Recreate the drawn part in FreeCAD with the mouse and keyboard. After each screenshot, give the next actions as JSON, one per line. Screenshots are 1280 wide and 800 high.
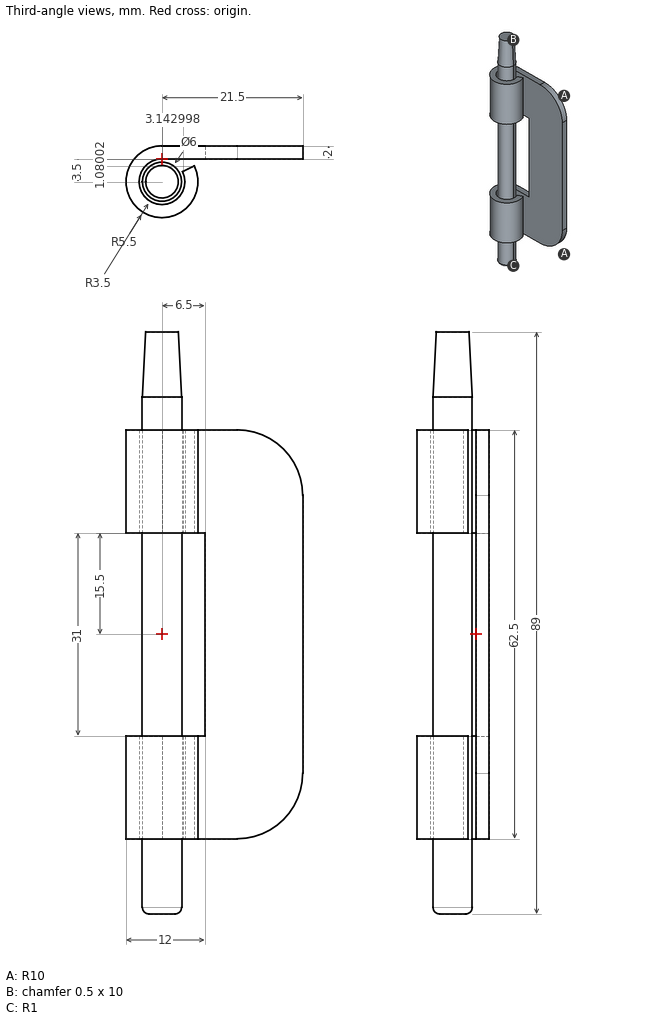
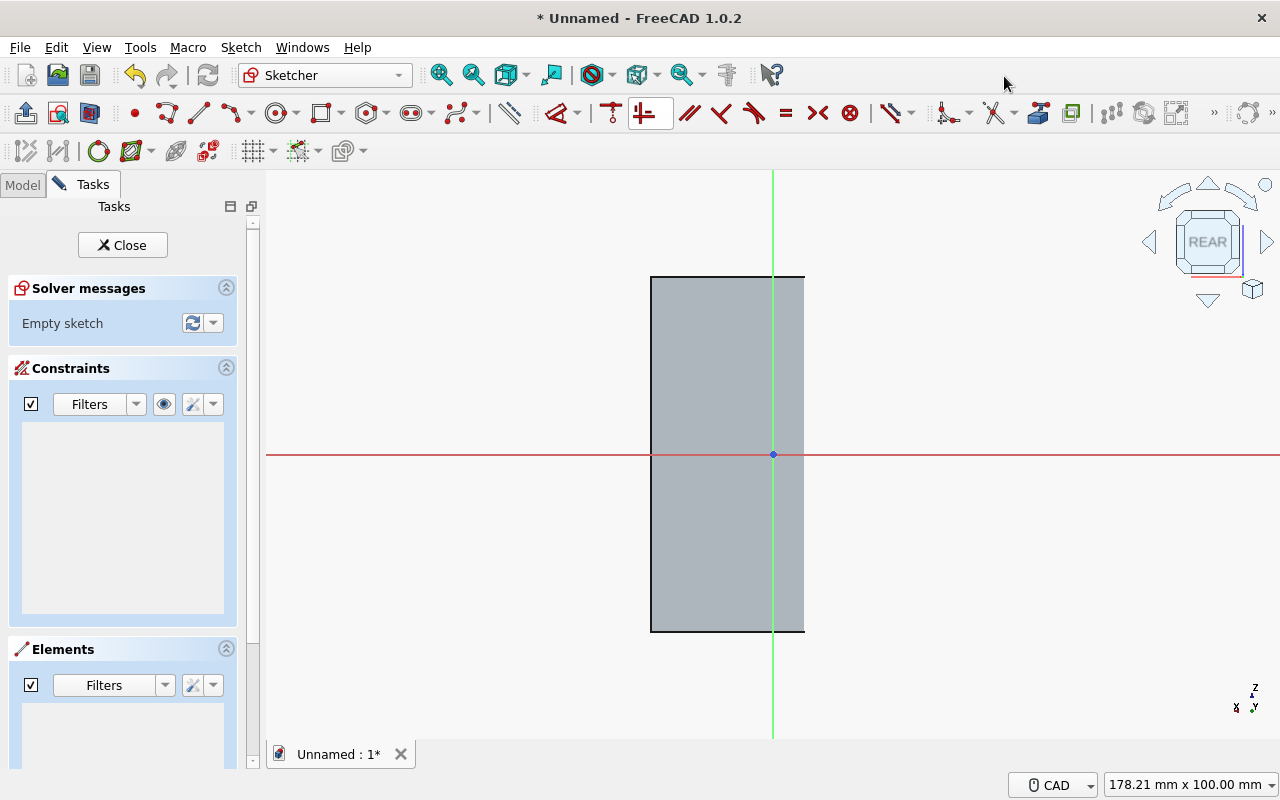
{"action": "scroll", "coordinate": [824, 454], "scroll_direction": "up", "scroll_amount": 4}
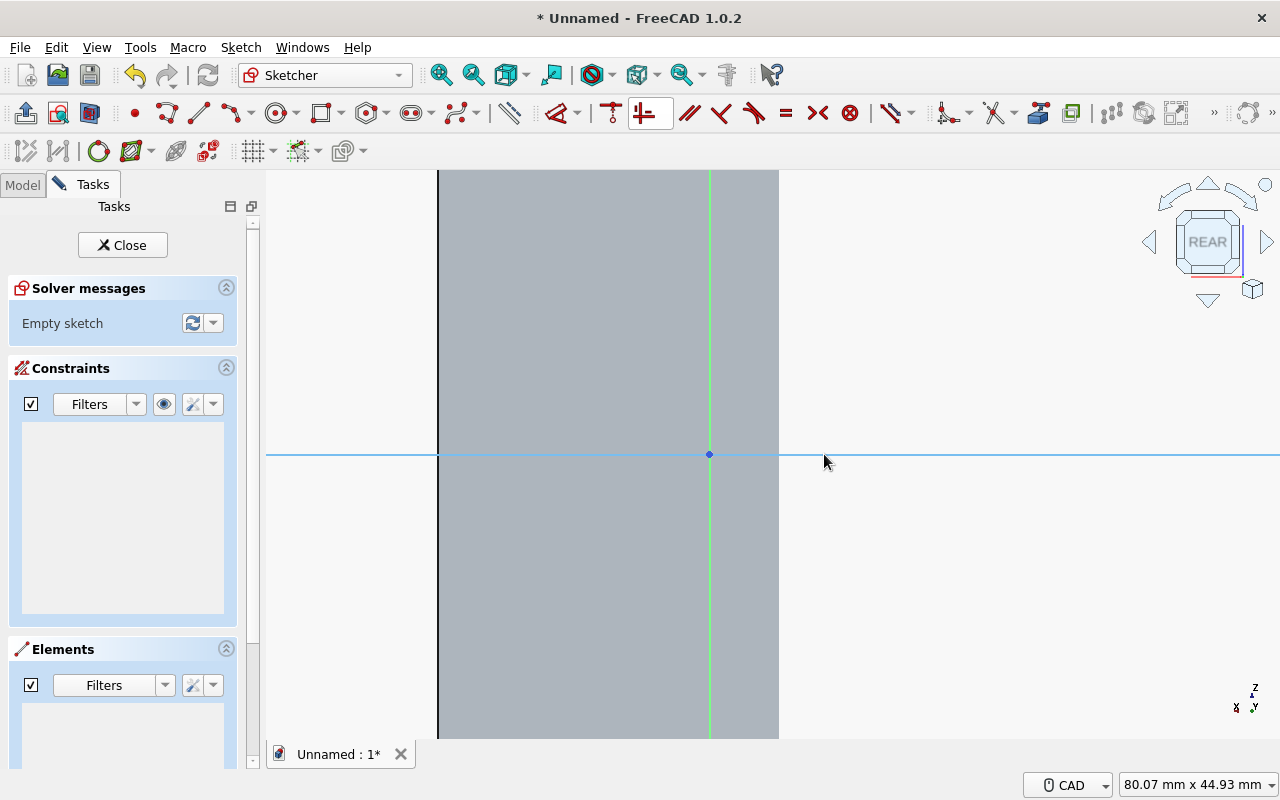
{"action": "key", "text": "g r"}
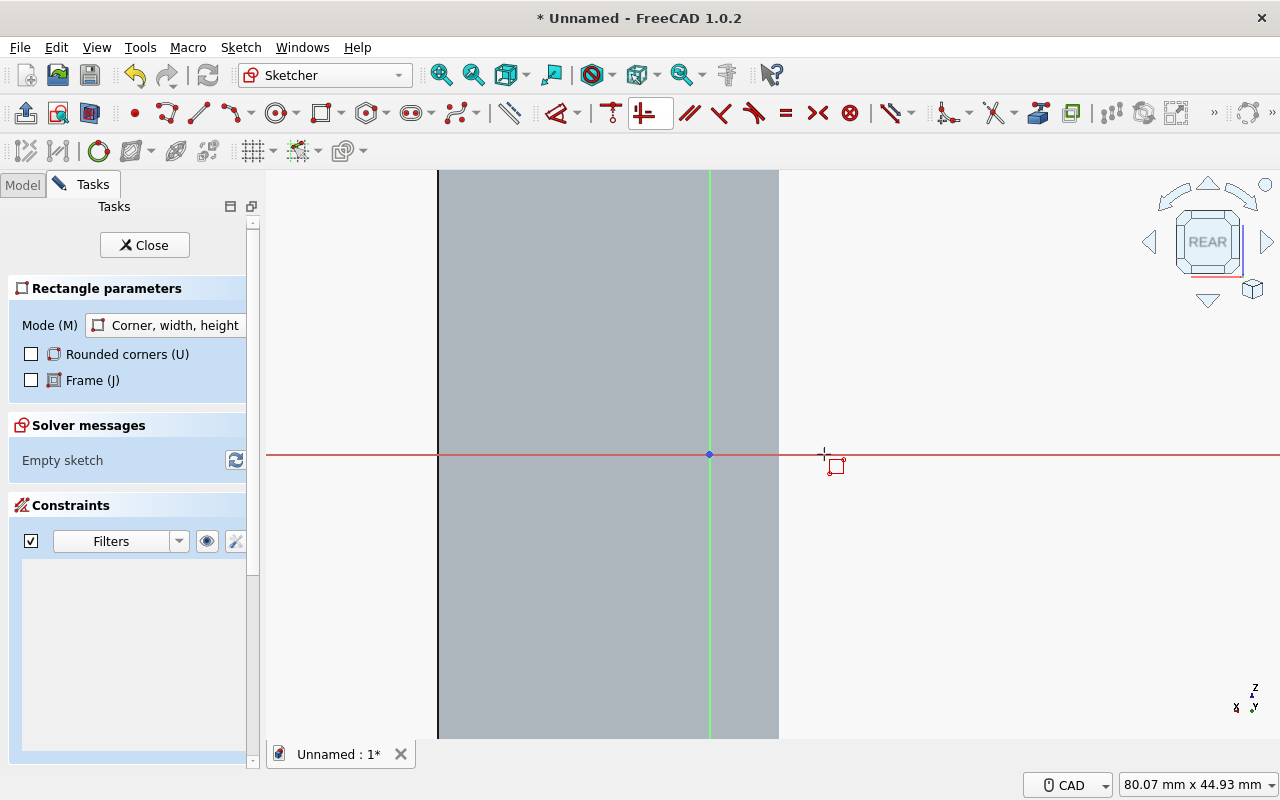
{"action": "left_click", "coordinate": [628, 258]}
{"action": "mouse_move", "coordinate": [779, 651]}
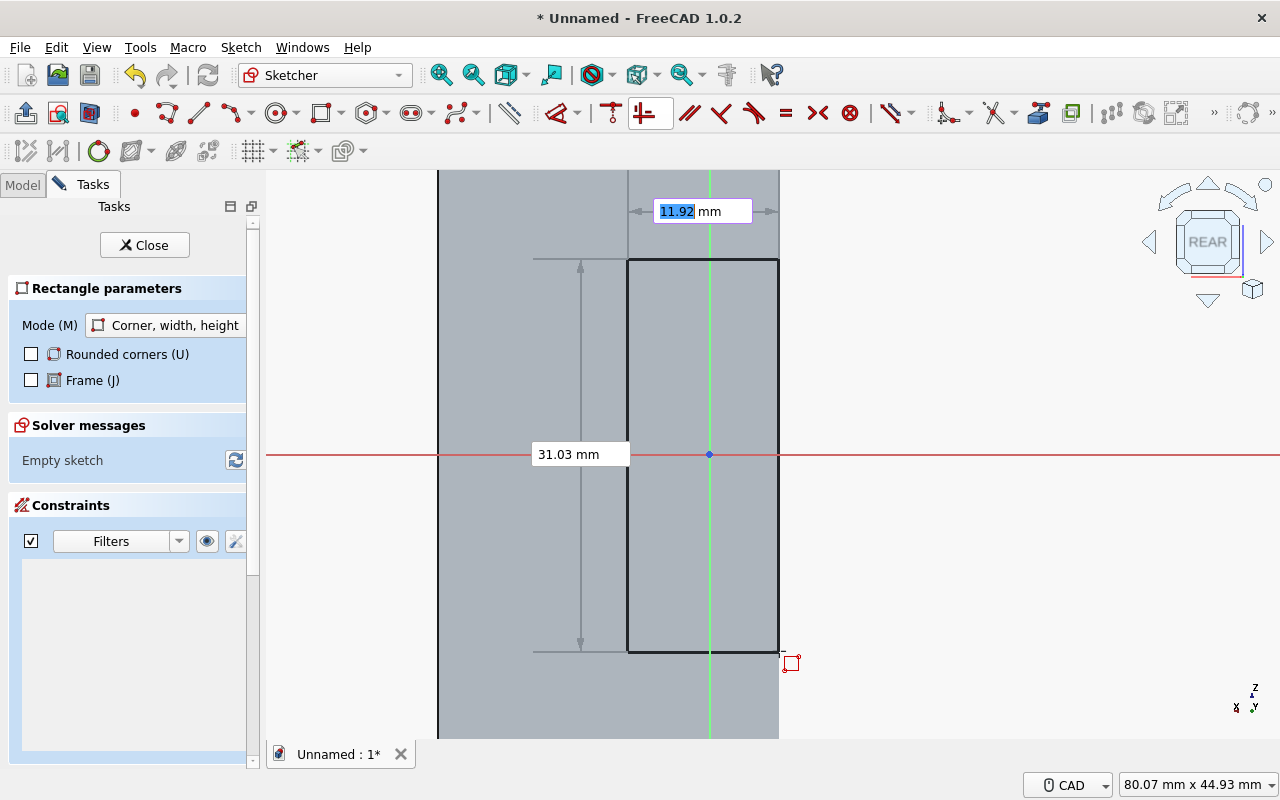
{"action": "type", "text": "12"}
{"action": "key", "text": "Tab"}
{"action": "type", "text": "31"}
{"action": "key", "text": "Return"}
{"action": "key", "text": "Escape"}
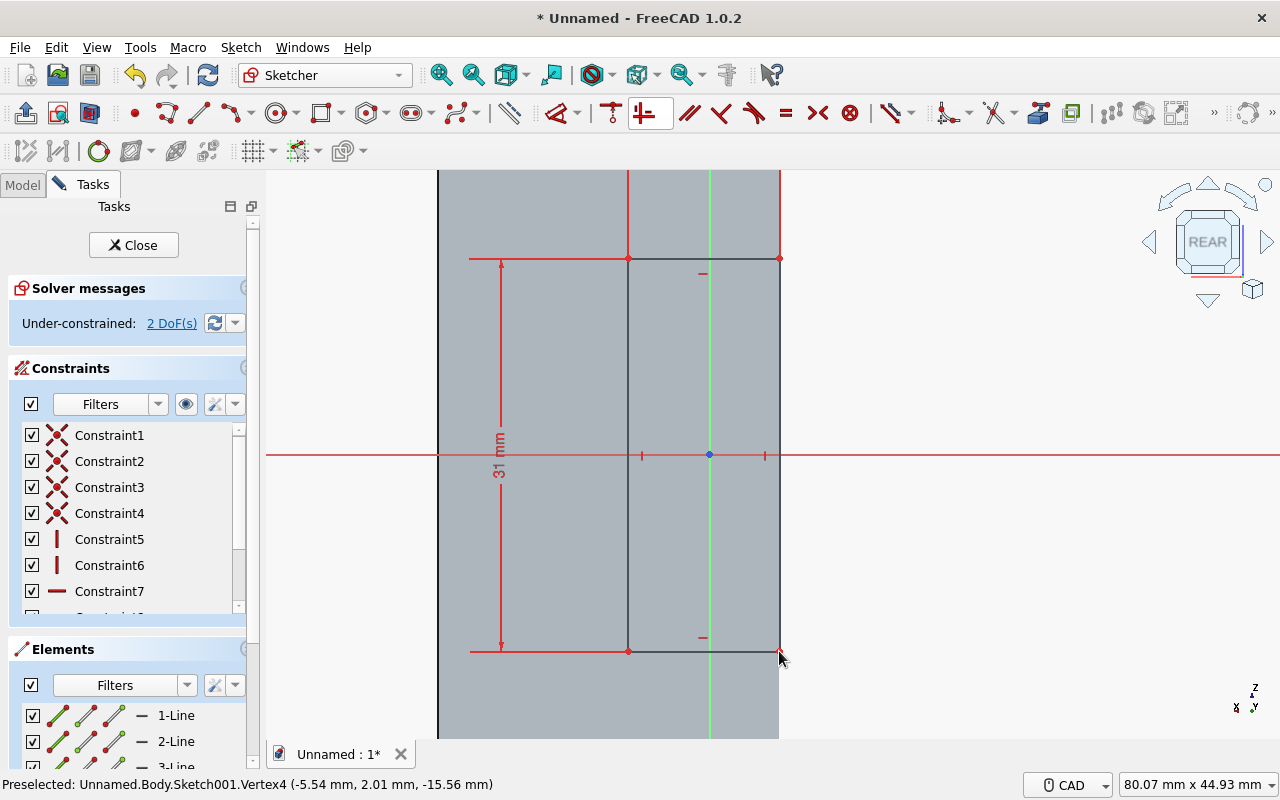
{"action": "left_click", "coordinate": [556, 114]}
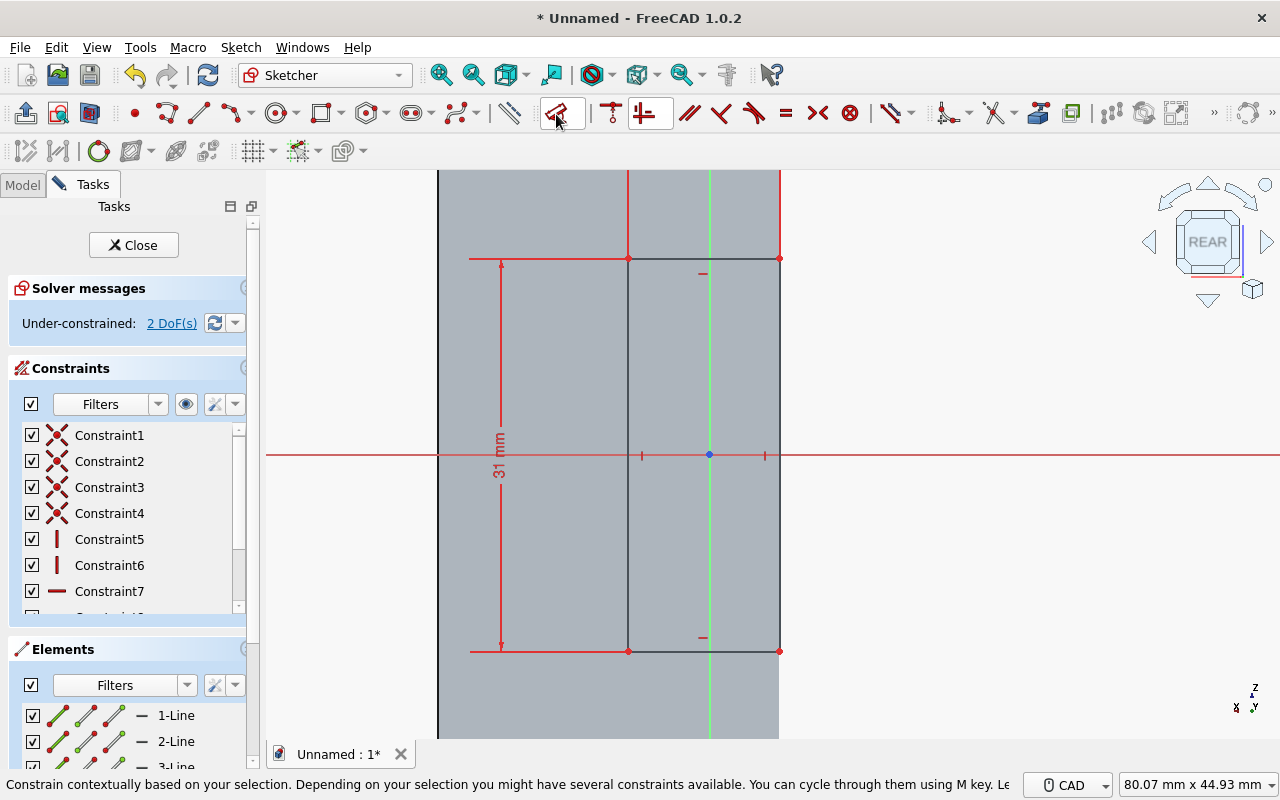
{"action": "left_click", "coordinate": [628, 259]}
{"action": "left_click", "coordinate": [669, 225]}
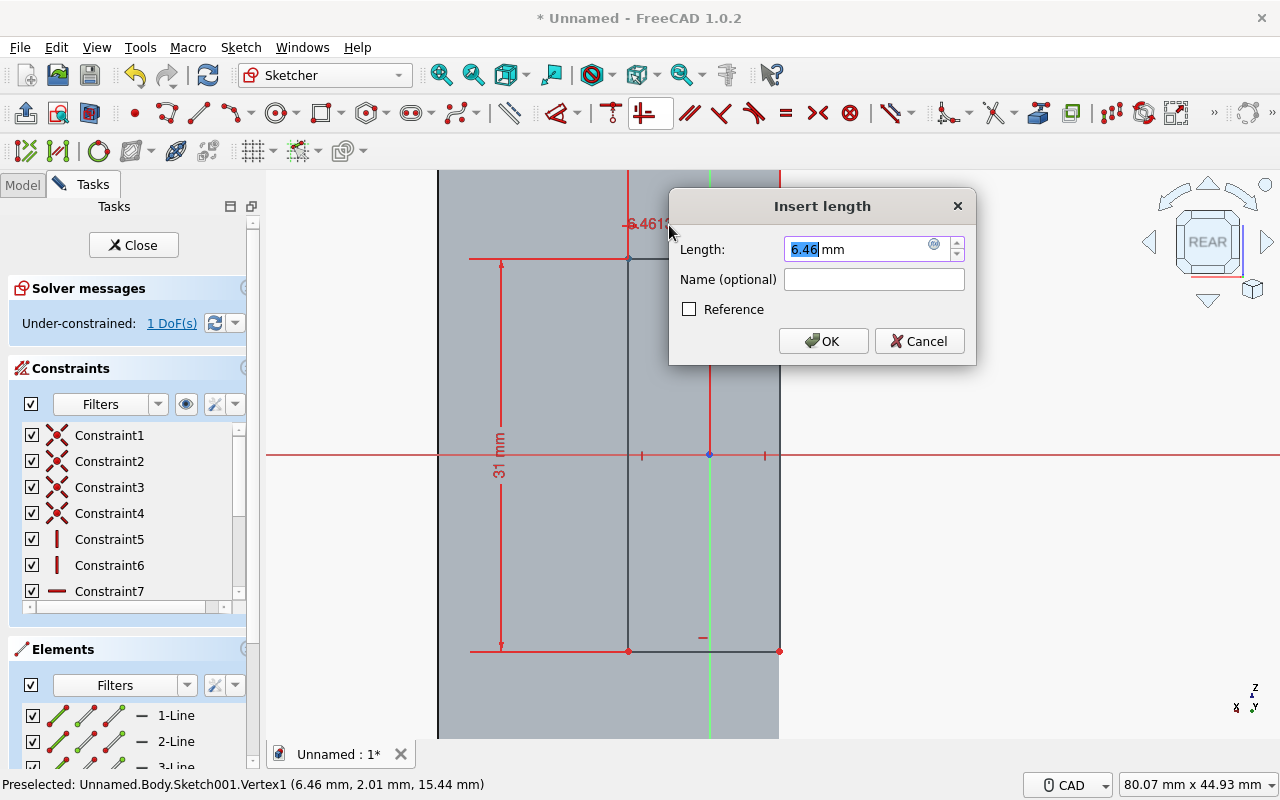
{"action": "type", "text": "6.5"}
{"action": "key", "text": "Return"}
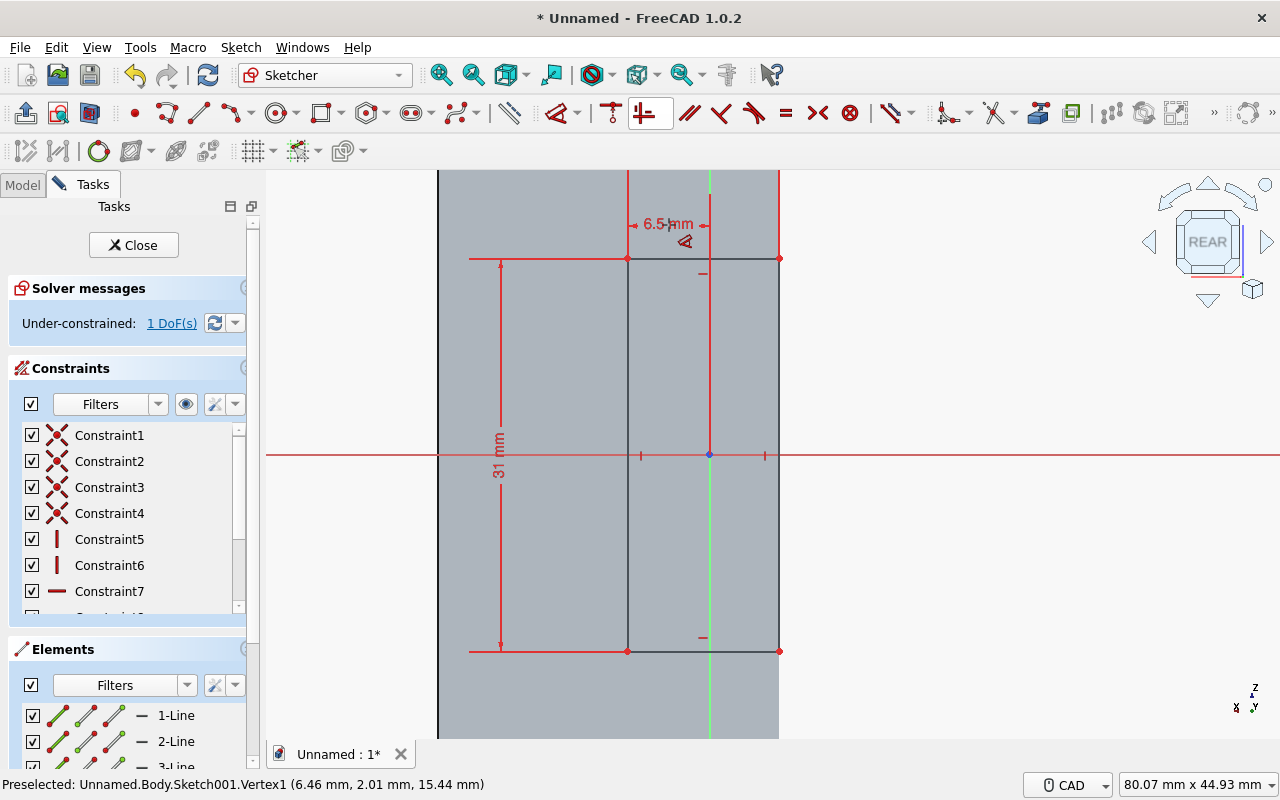
{"action": "left_click", "coordinate": [628, 259]}
{"action": "left_click", "coordinate": [594, 357]}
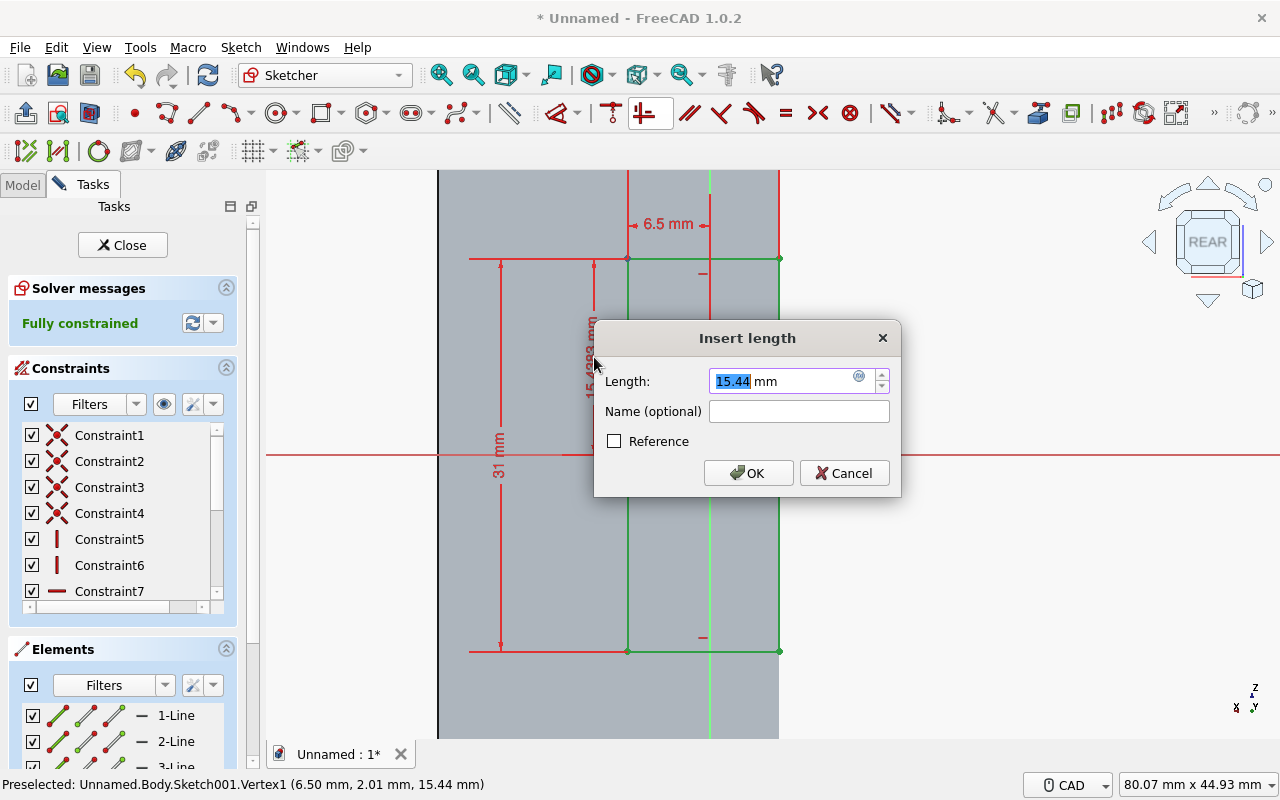
{"action": "type", "text": "15.5"}
{"action": "key", "text": "Return"}
{"action": "key", "text": "Escape"}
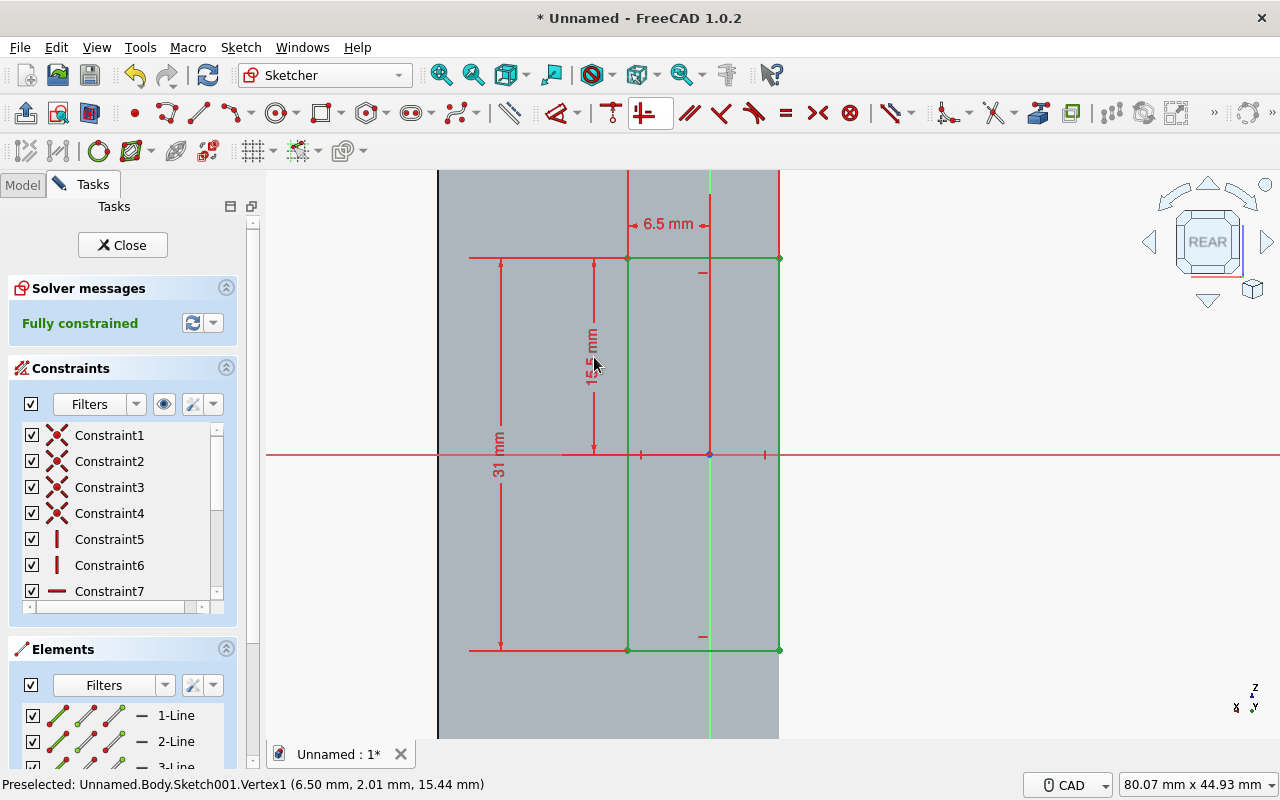
{"action": "left_click", "coordinate": [123, 245]}